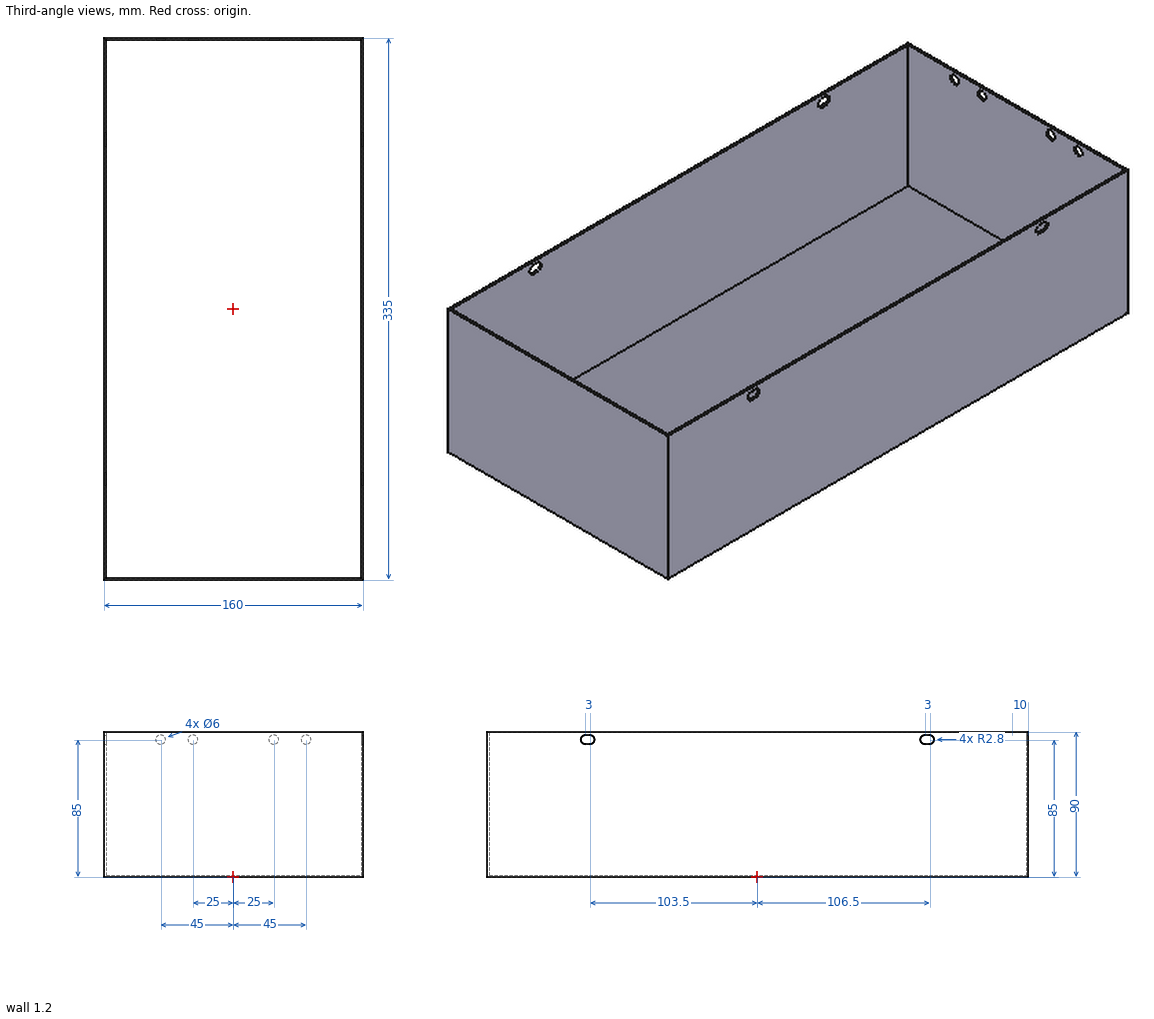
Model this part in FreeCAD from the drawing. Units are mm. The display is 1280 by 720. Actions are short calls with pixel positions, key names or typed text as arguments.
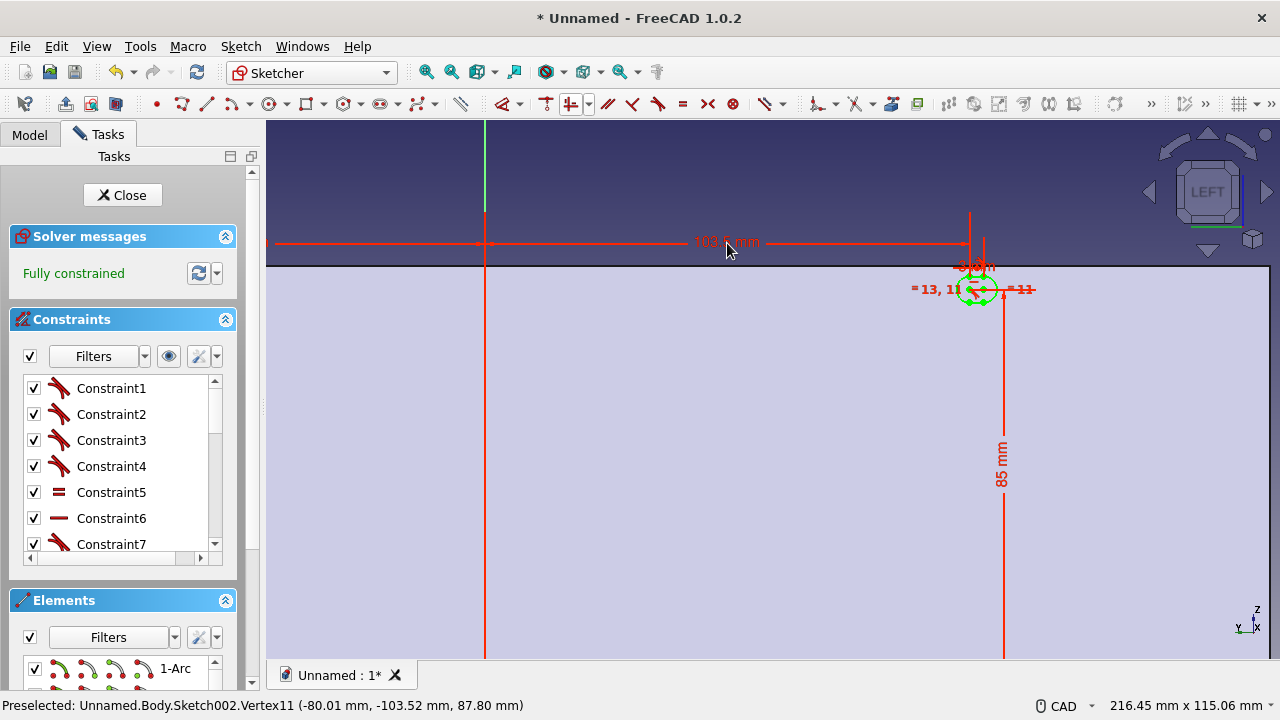
click(123, 195)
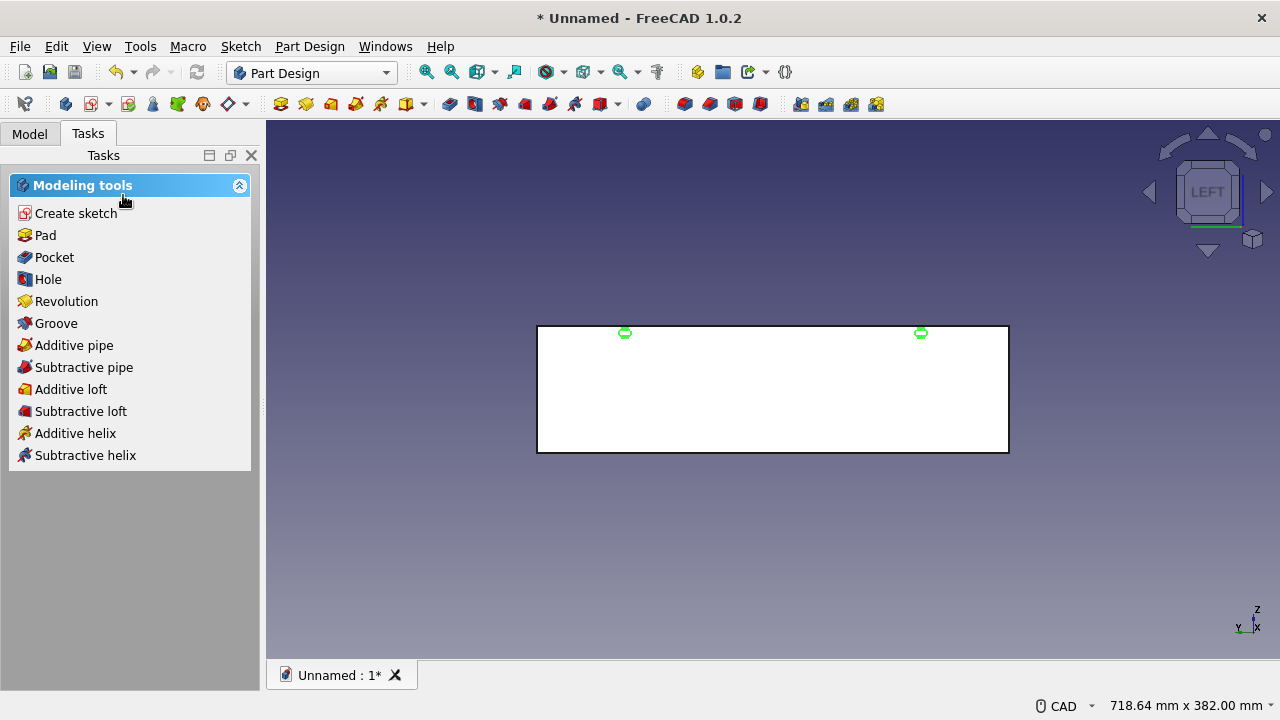
click(450, 104)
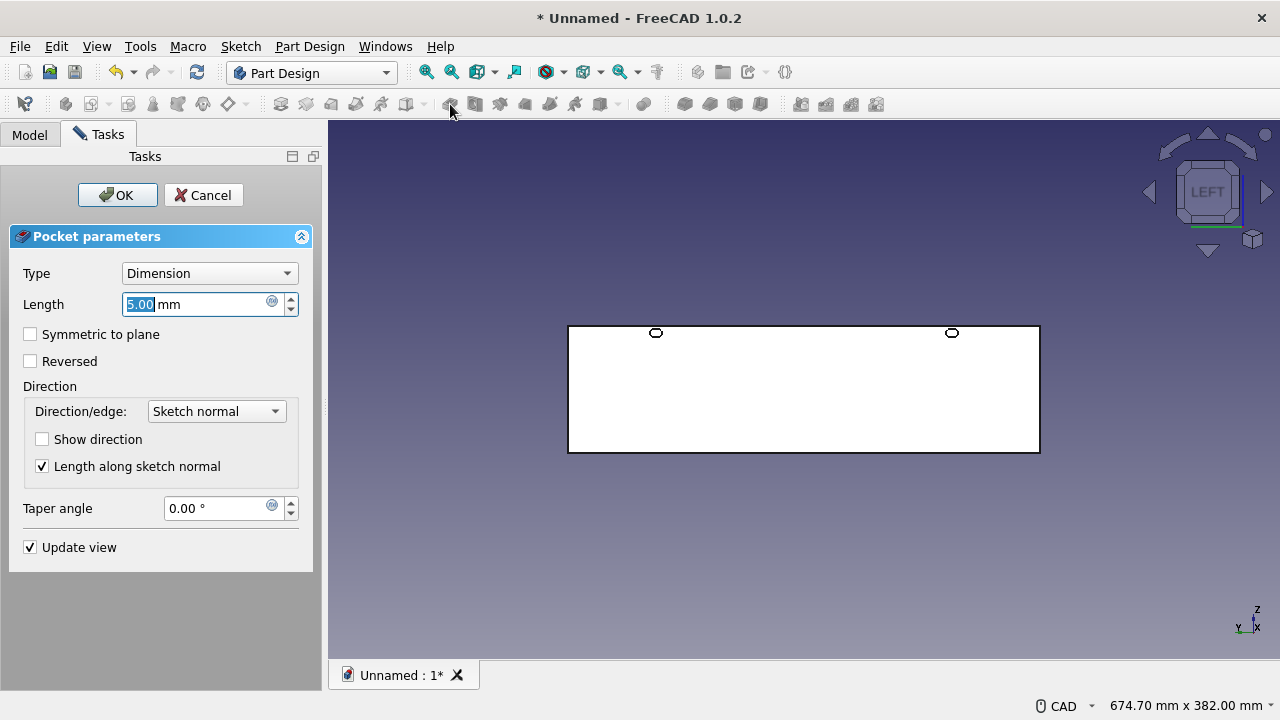
click(210, 274)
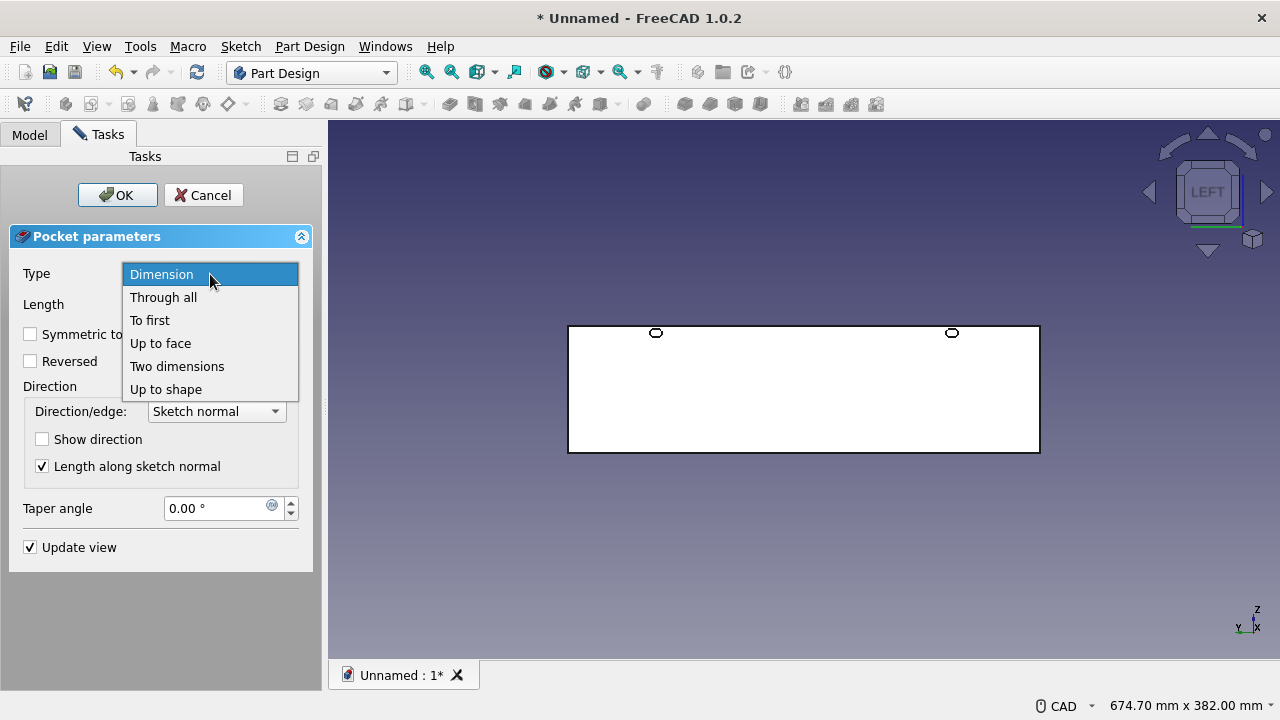
click(208, 298)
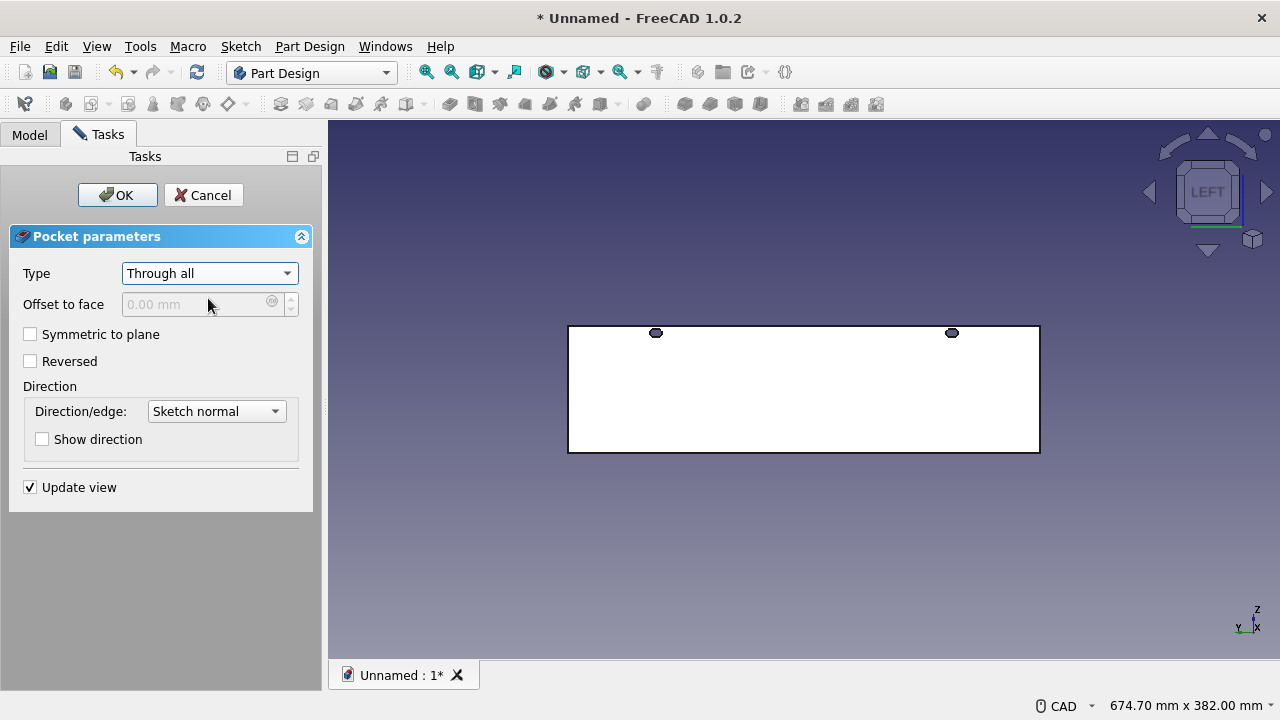
click(118, 195)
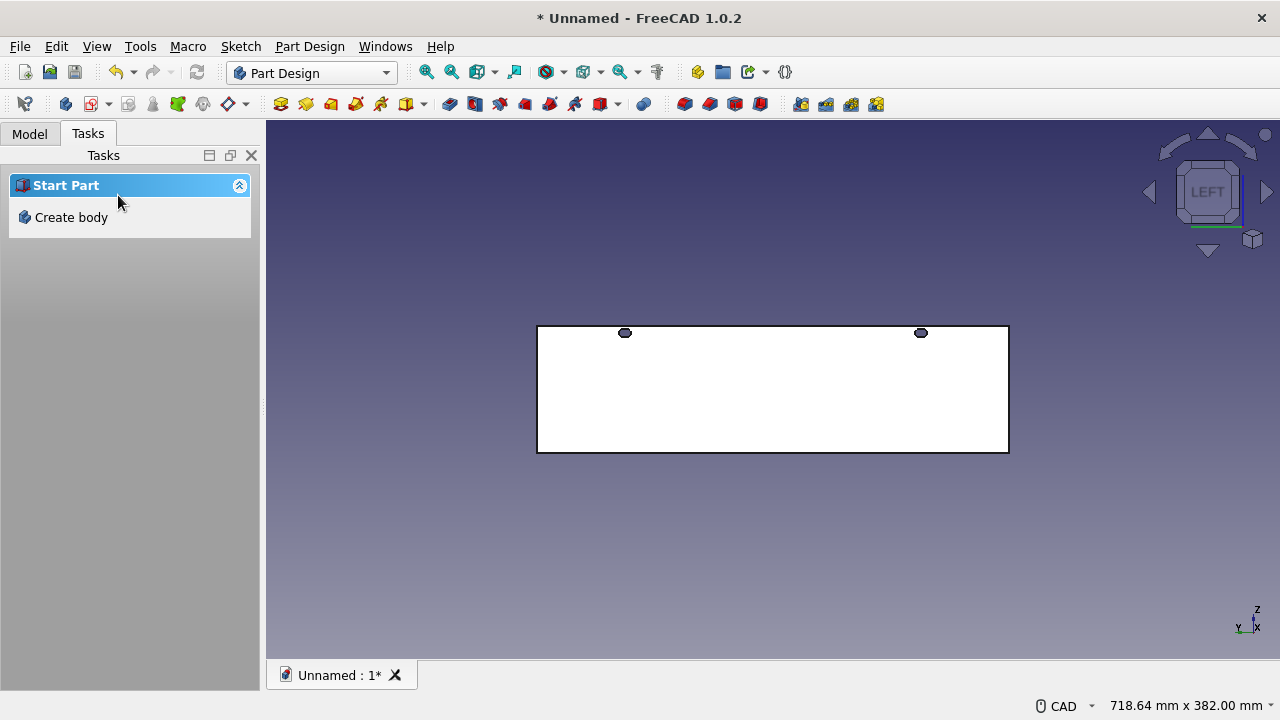
key(0)